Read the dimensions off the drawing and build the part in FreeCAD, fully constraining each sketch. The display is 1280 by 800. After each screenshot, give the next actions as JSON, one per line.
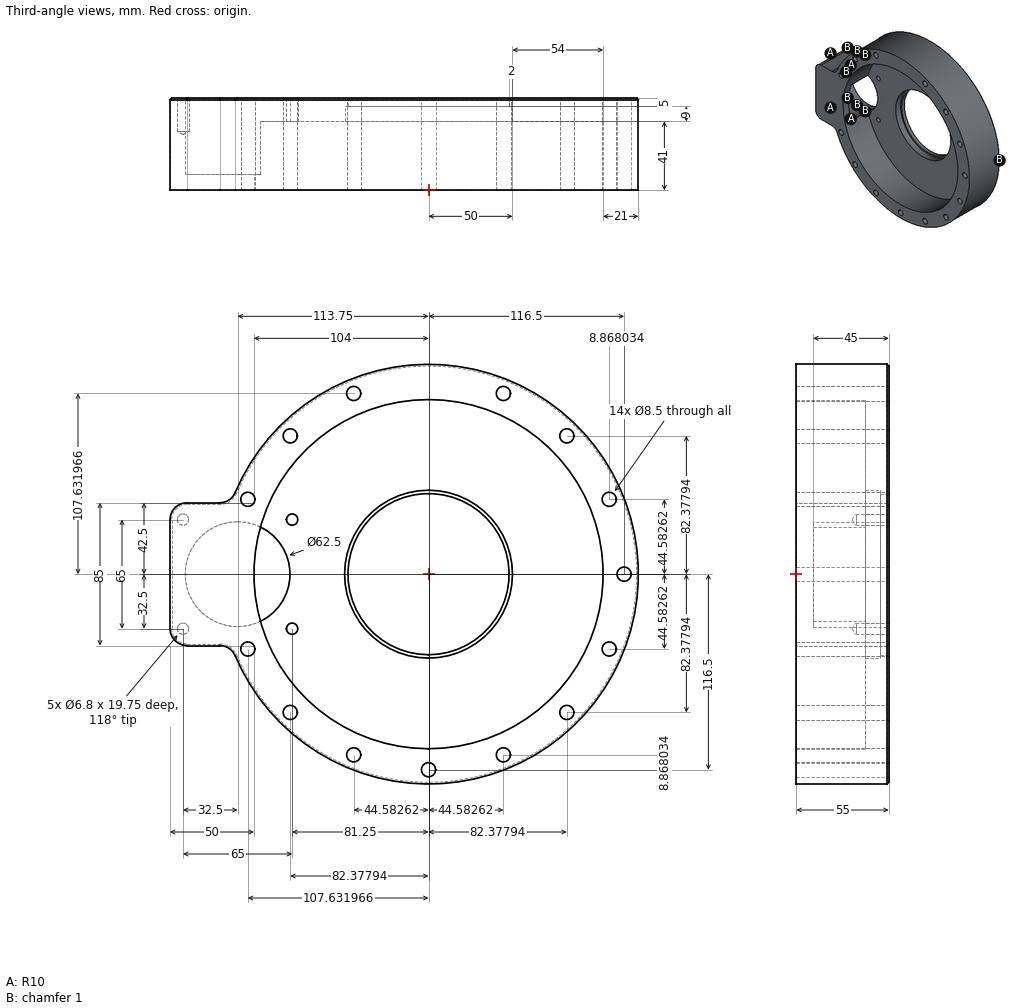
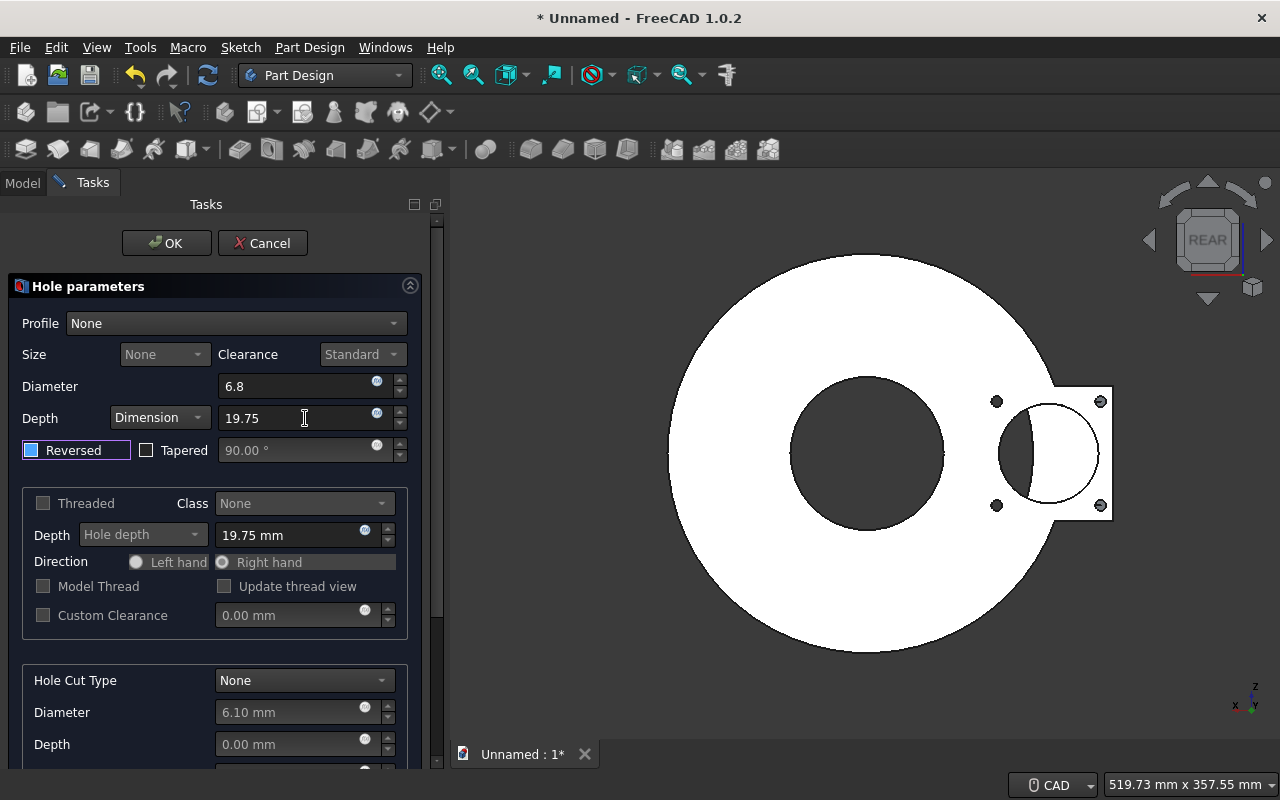
{"action": "left_click", "coordinate": [167, 243]}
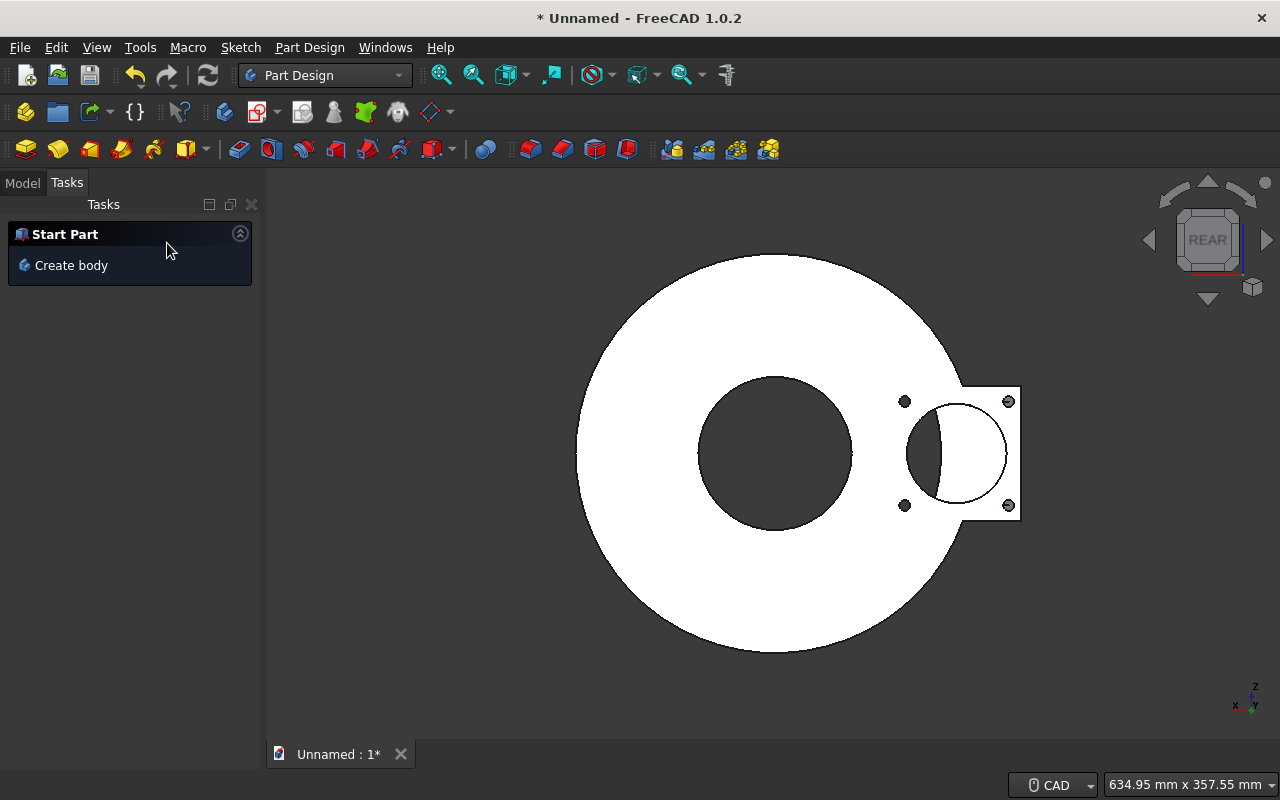
{"action": "key", "text": "0"}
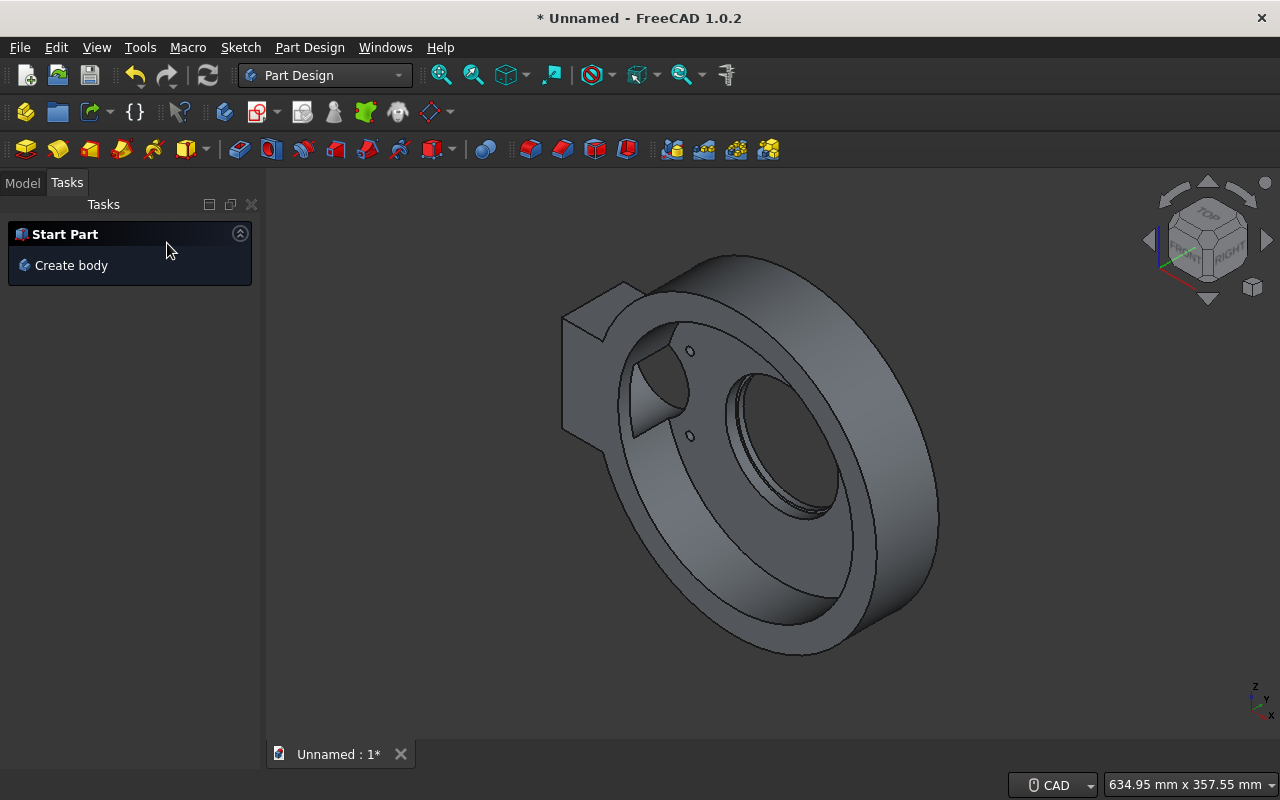
{"action": "key", "text": "2"}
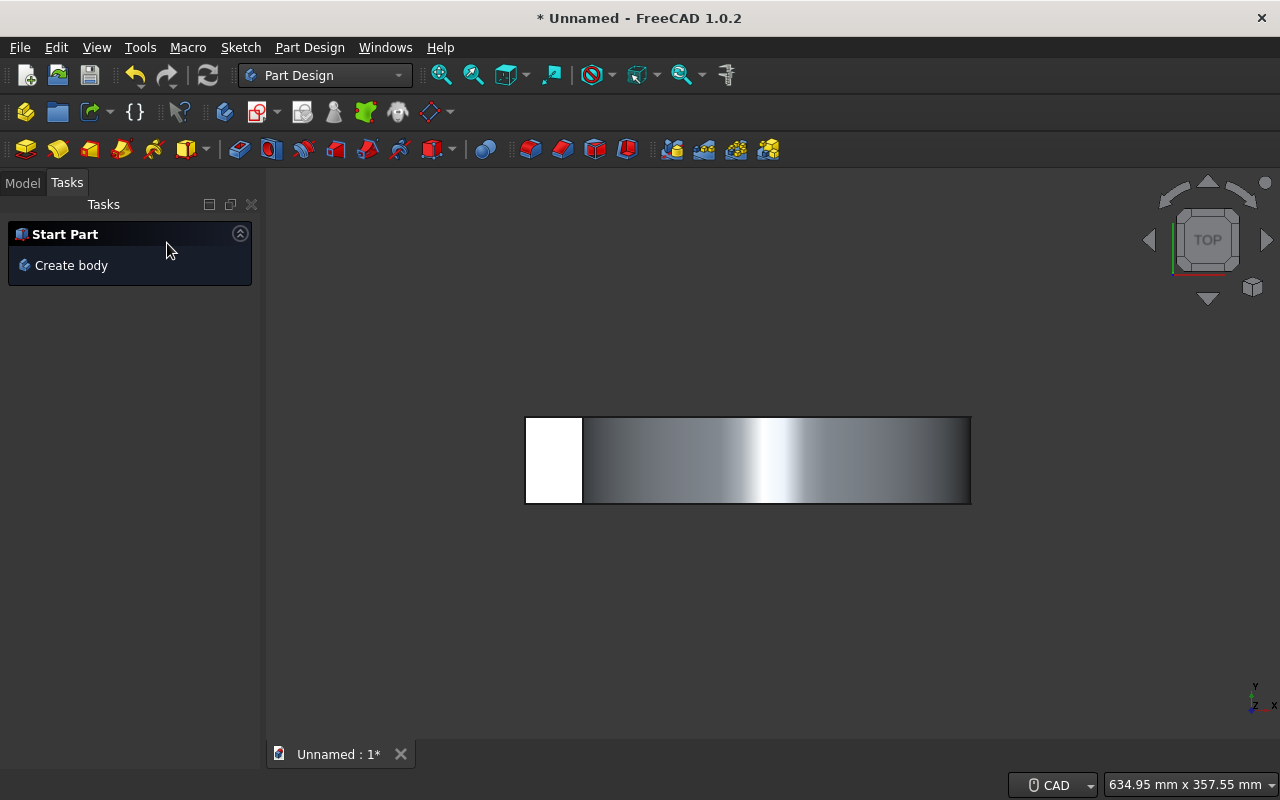
{"action": "left_click", "coordinate": [442, 76]}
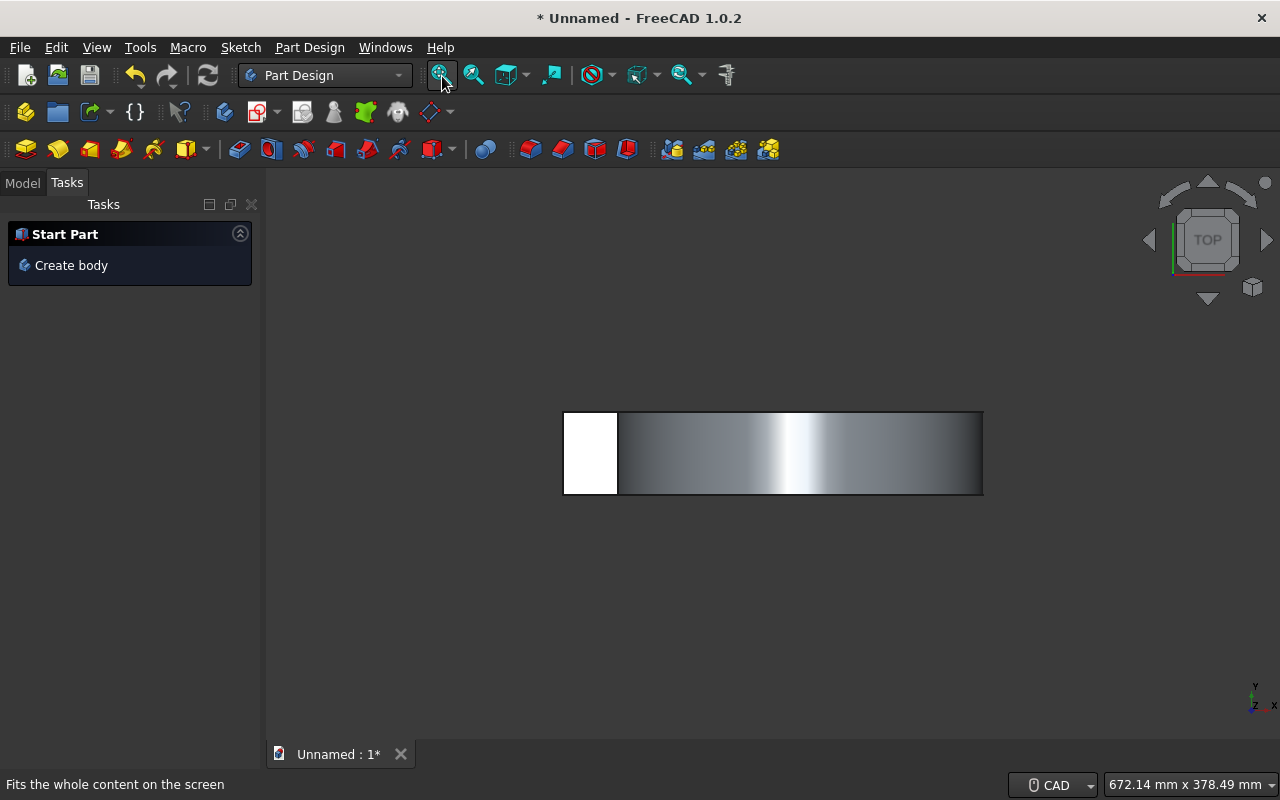
{"action": "left_click", "coordinate": [563, 452]}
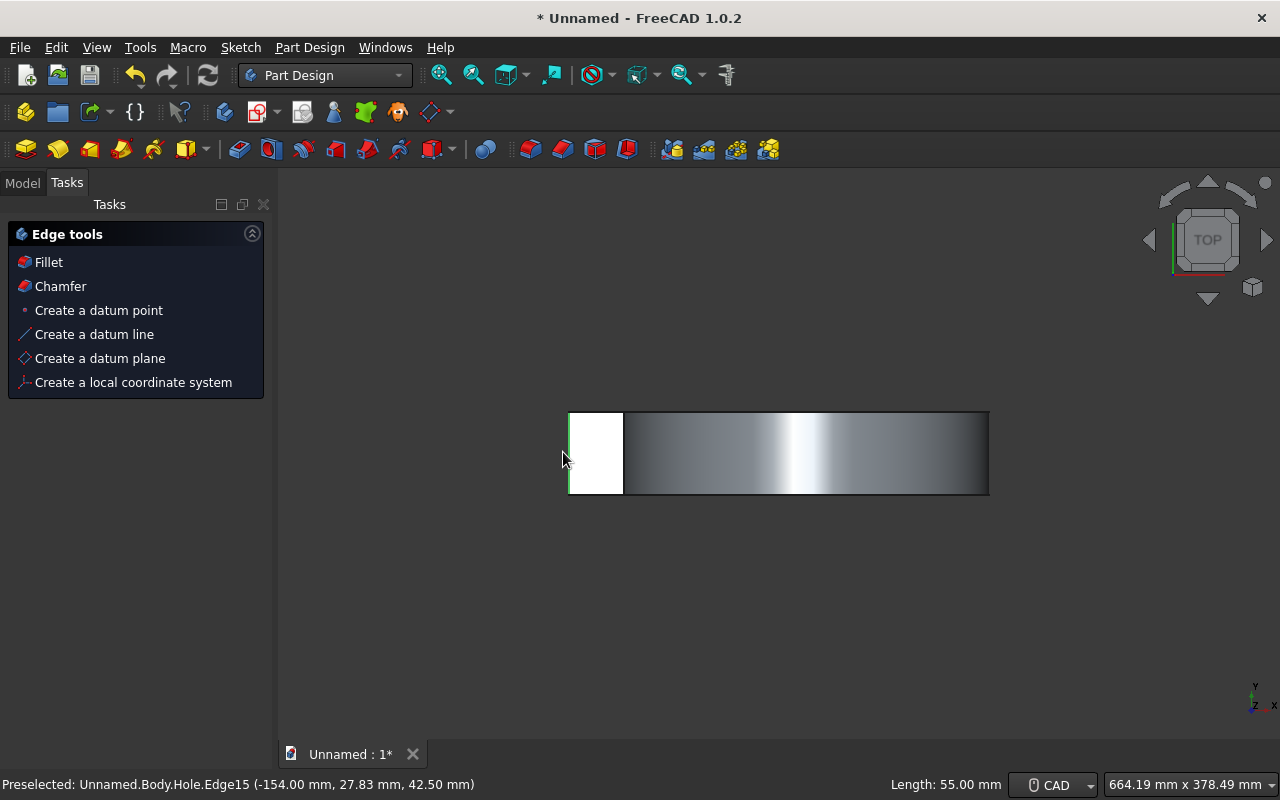
{"action": "key", "text": "1"}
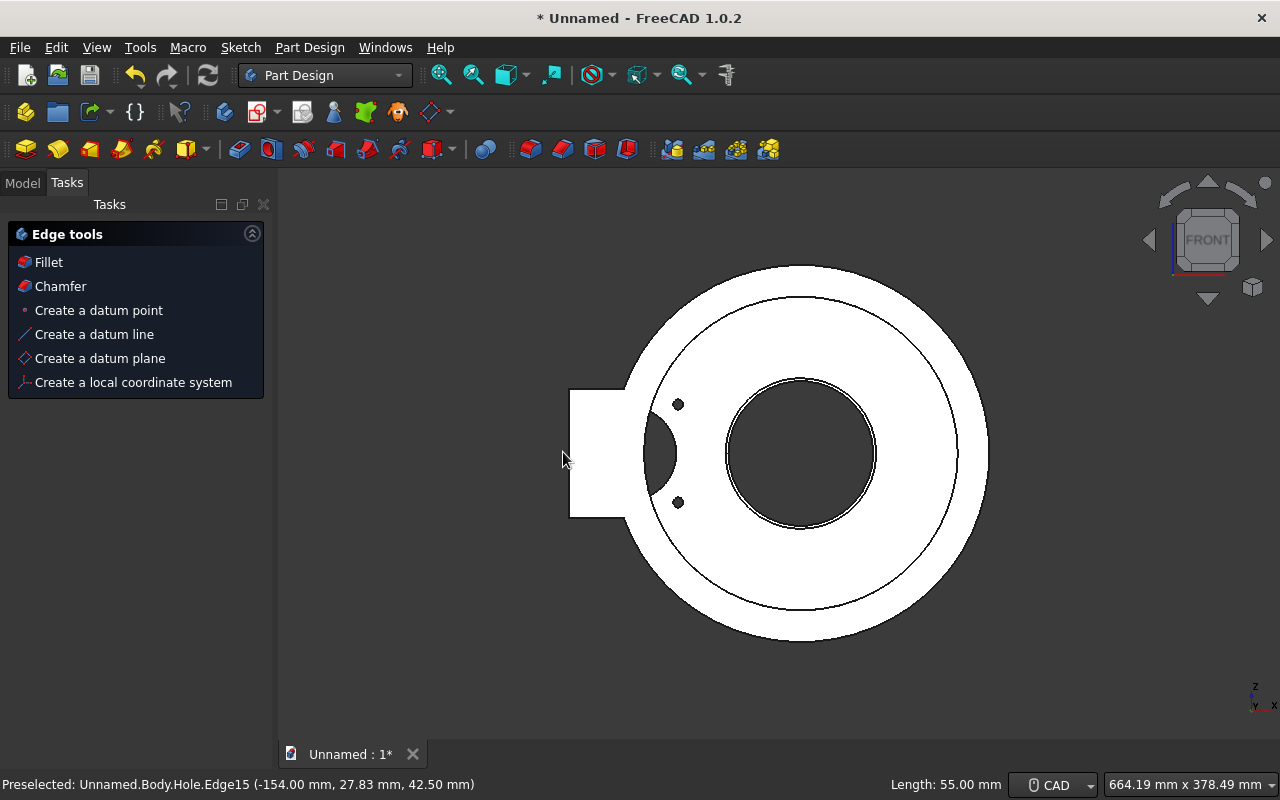
{"action": "key", "text": "3"}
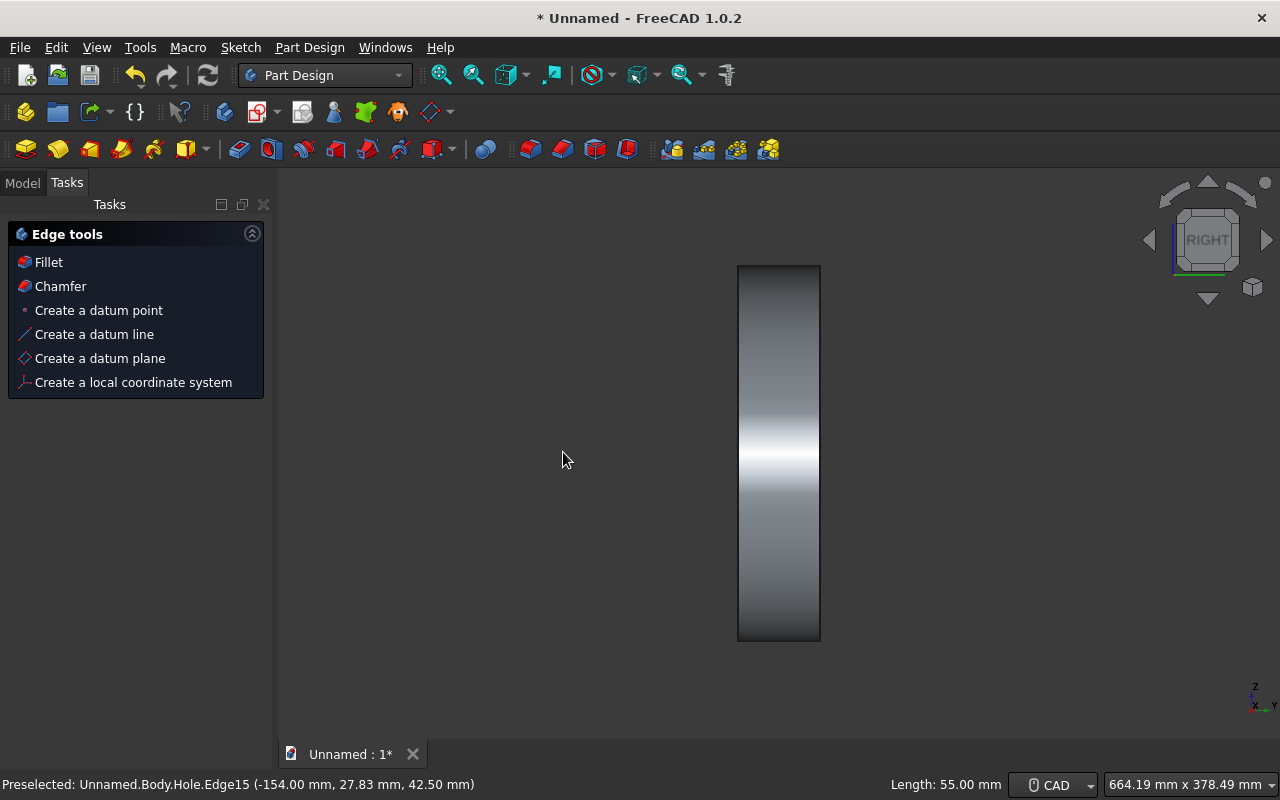
{"action": "key", "text": "5"}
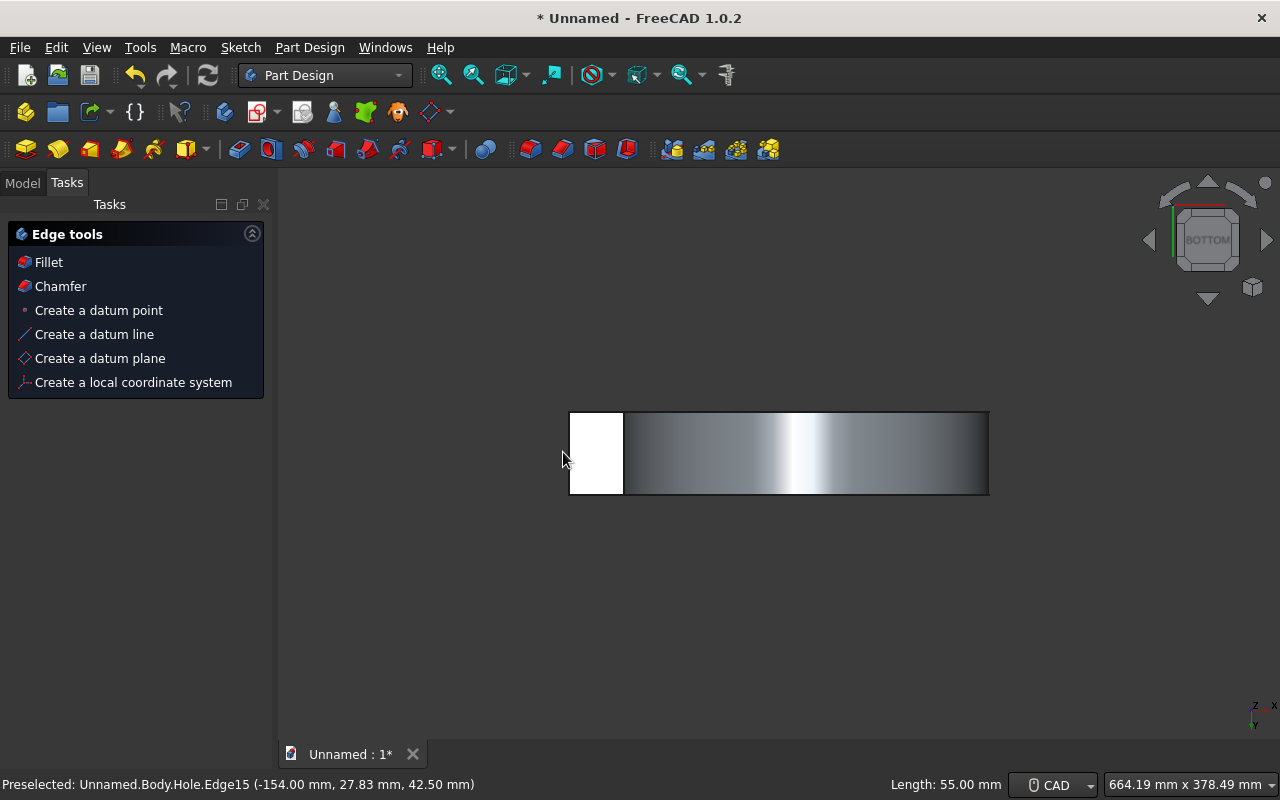
{"action": "left_click", "coordinate": [442, 76]}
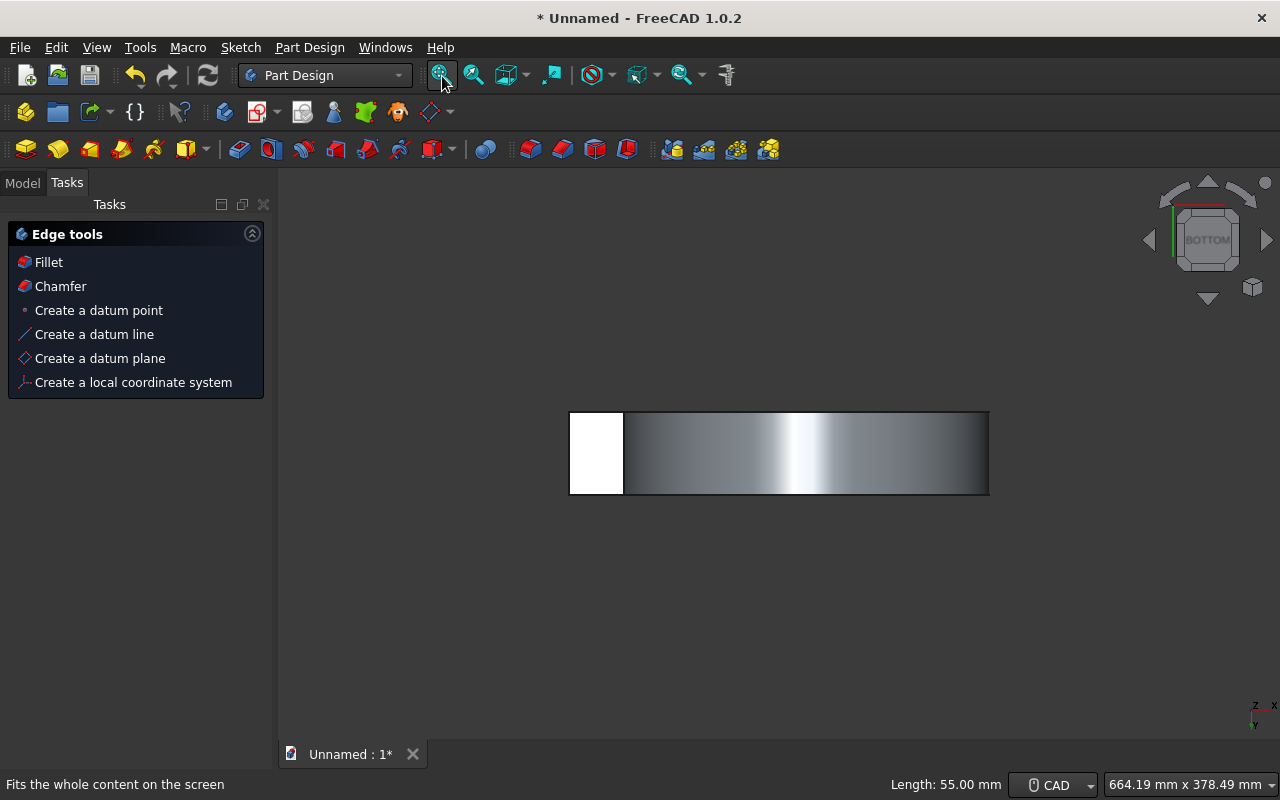
{"action": "left_click", "coordinate": [569, 452], "text": "ctrl"}